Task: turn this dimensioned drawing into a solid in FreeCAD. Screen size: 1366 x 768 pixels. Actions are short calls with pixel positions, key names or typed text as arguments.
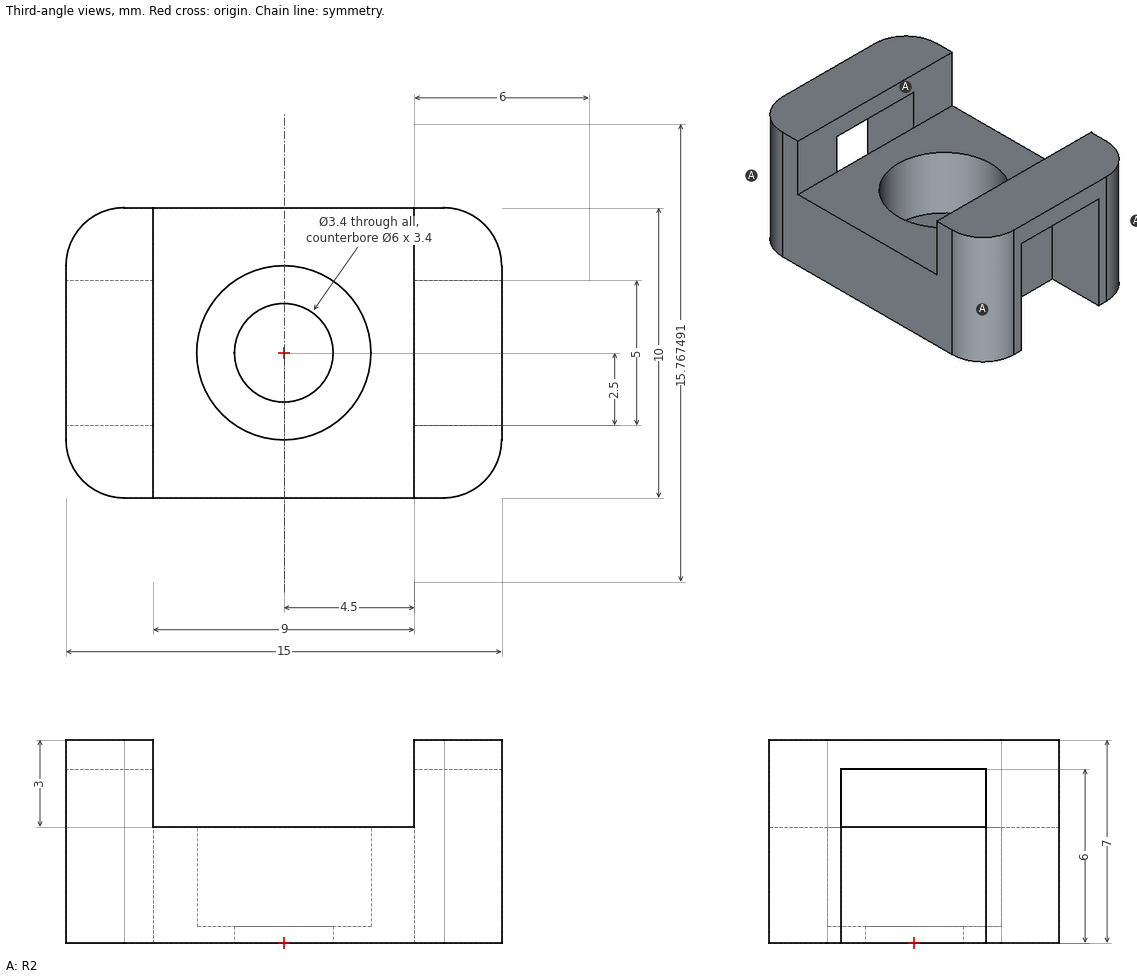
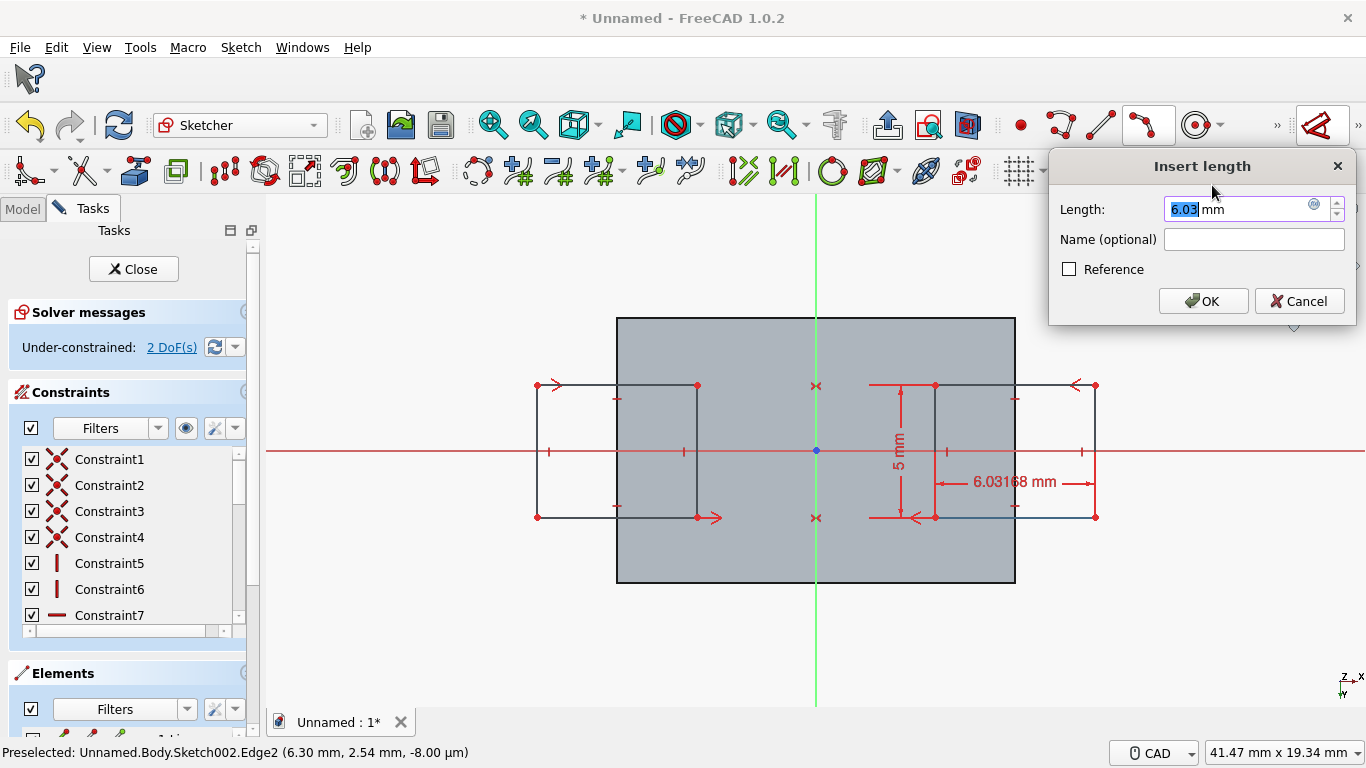
text(6)
key(Return)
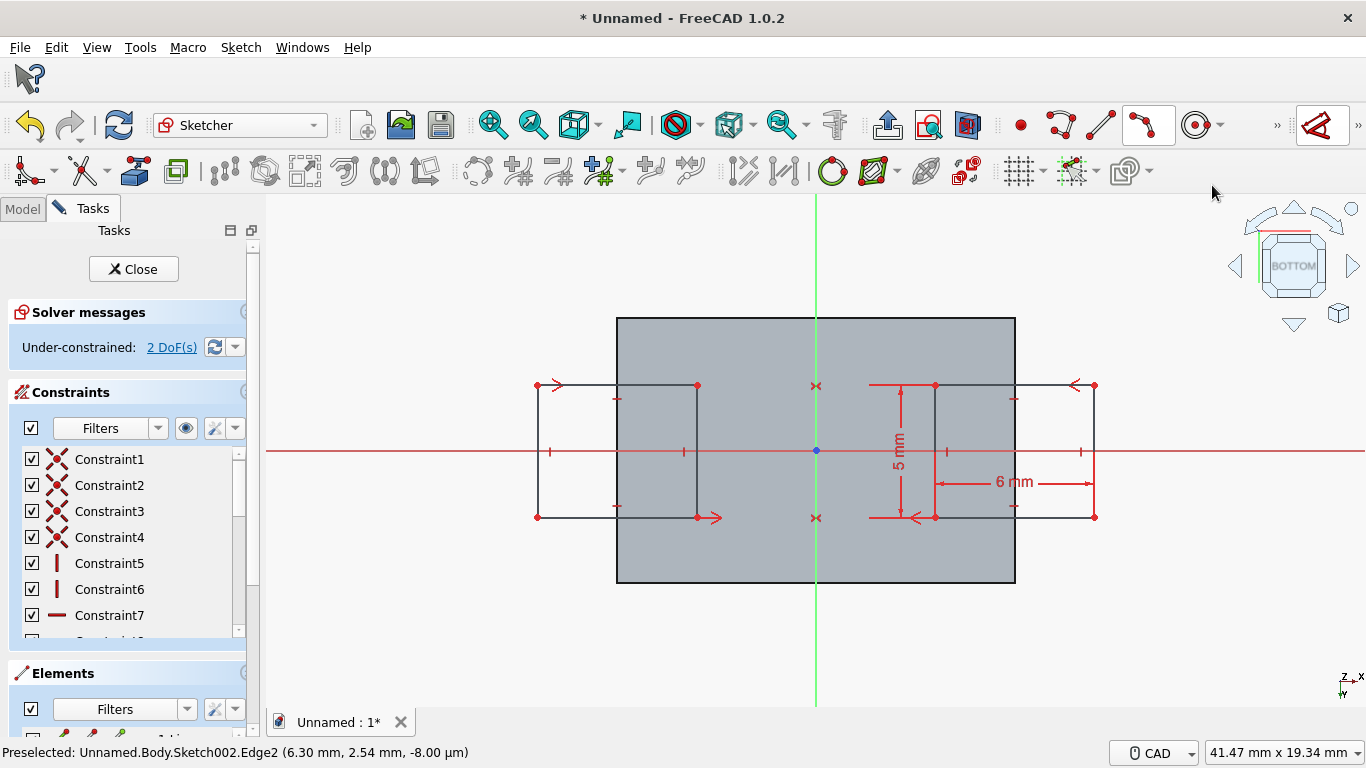
click(935, 385)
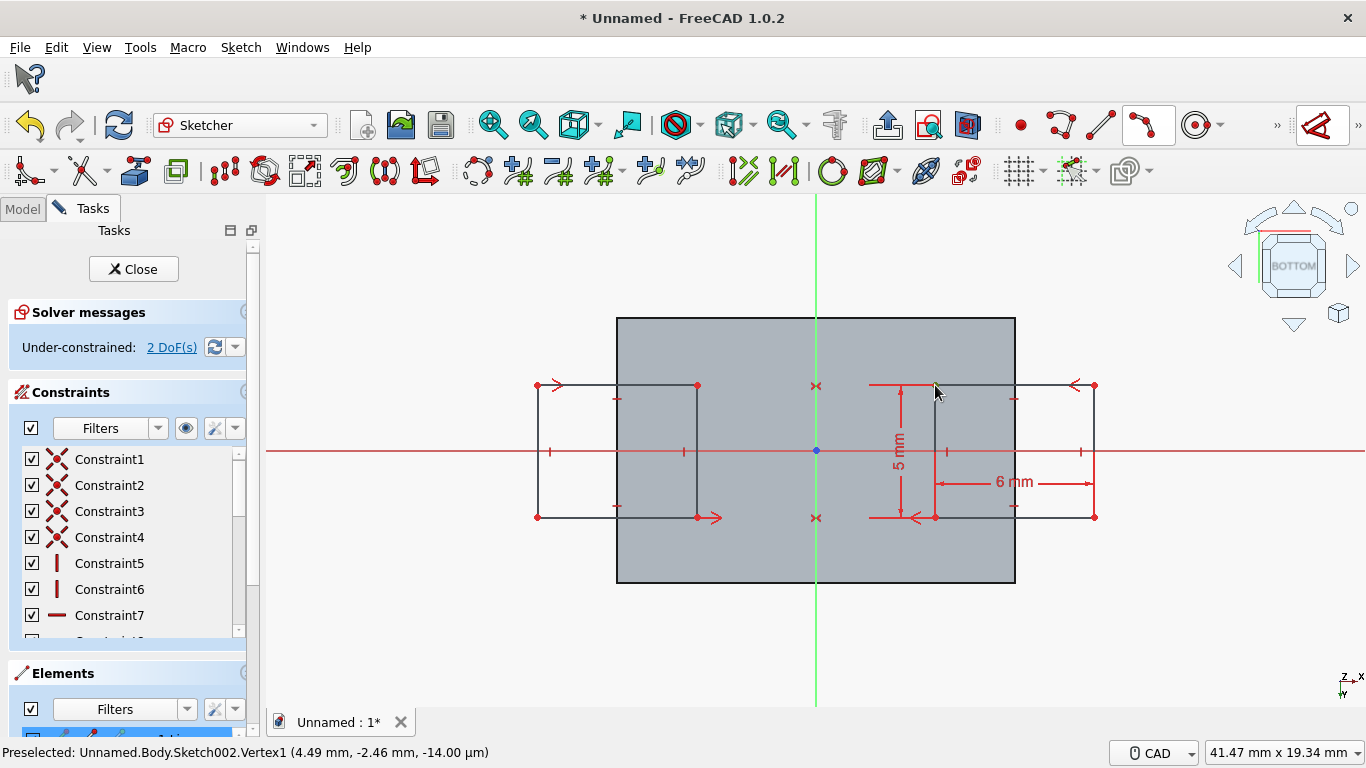
key(l)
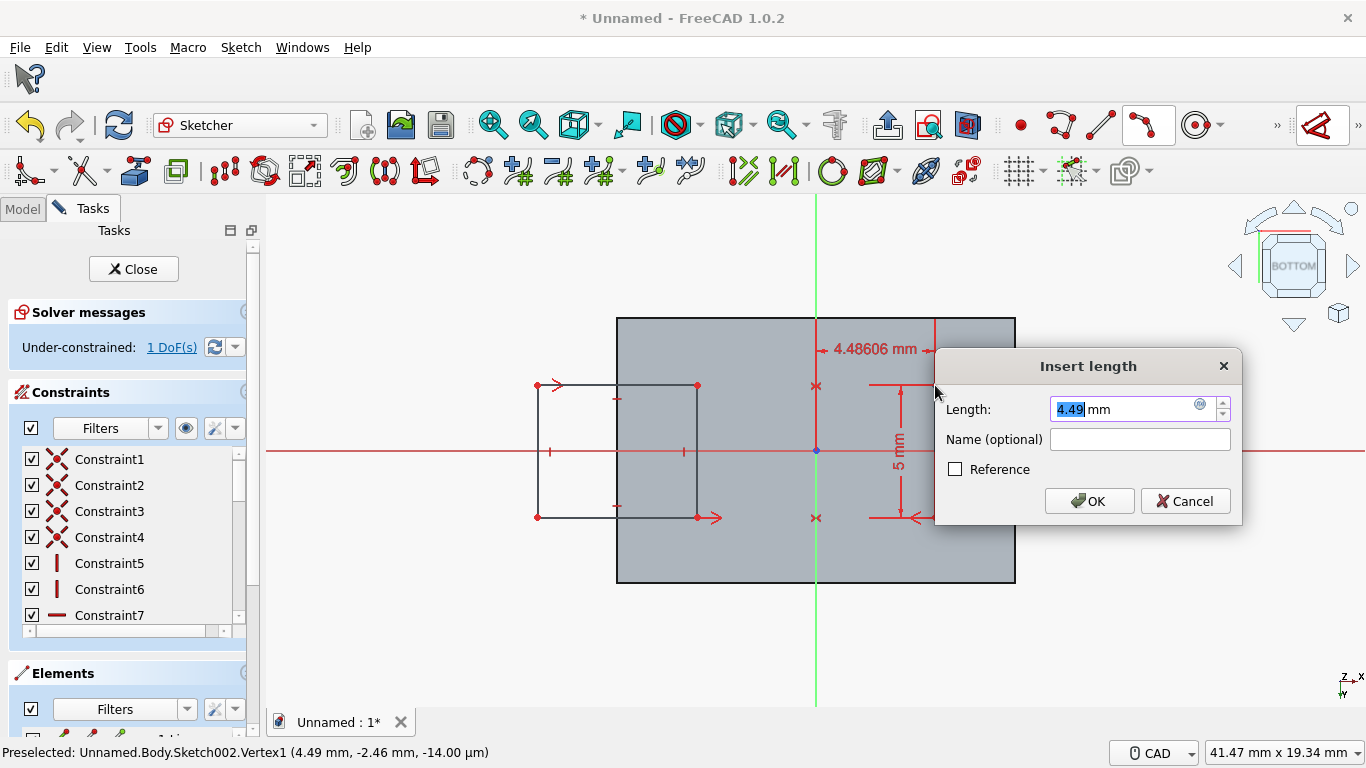
text(4.5)
key(Return)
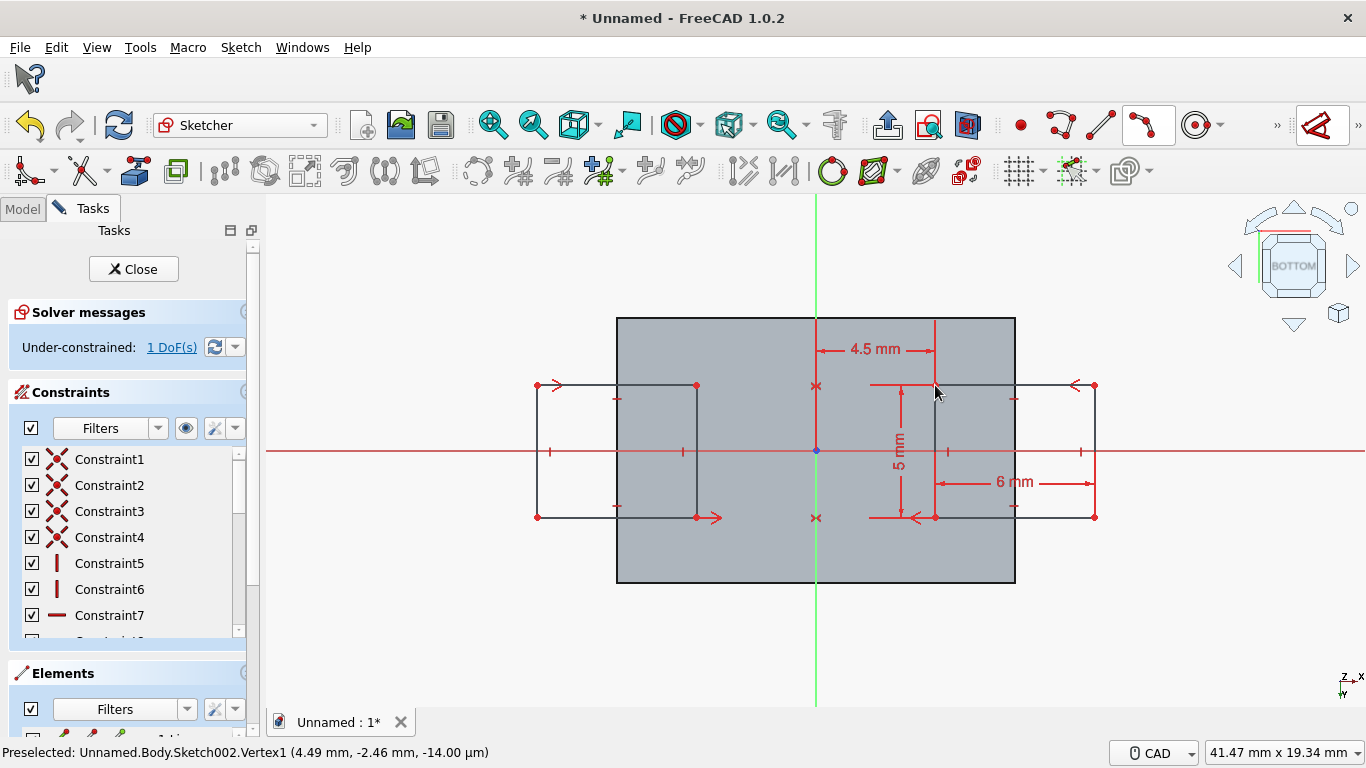
click(935, 385)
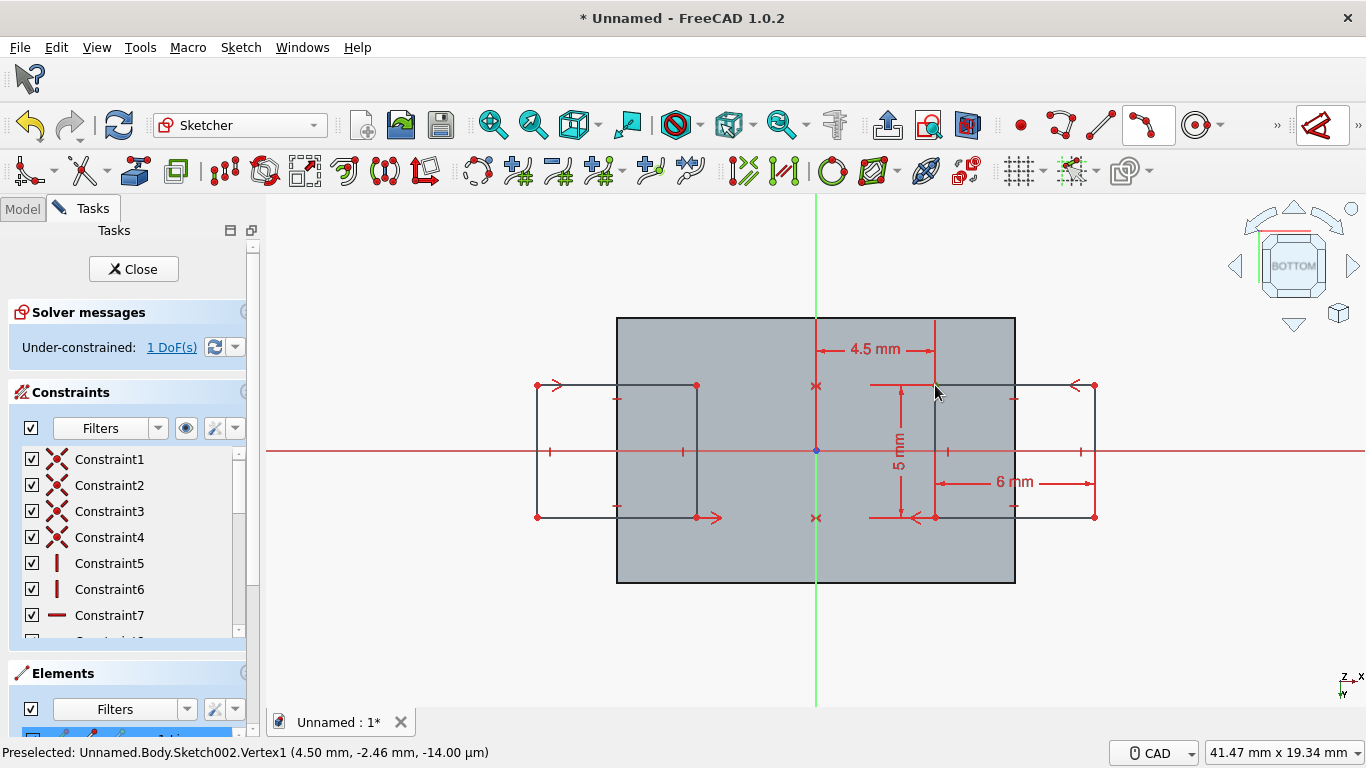
click(1344, 126)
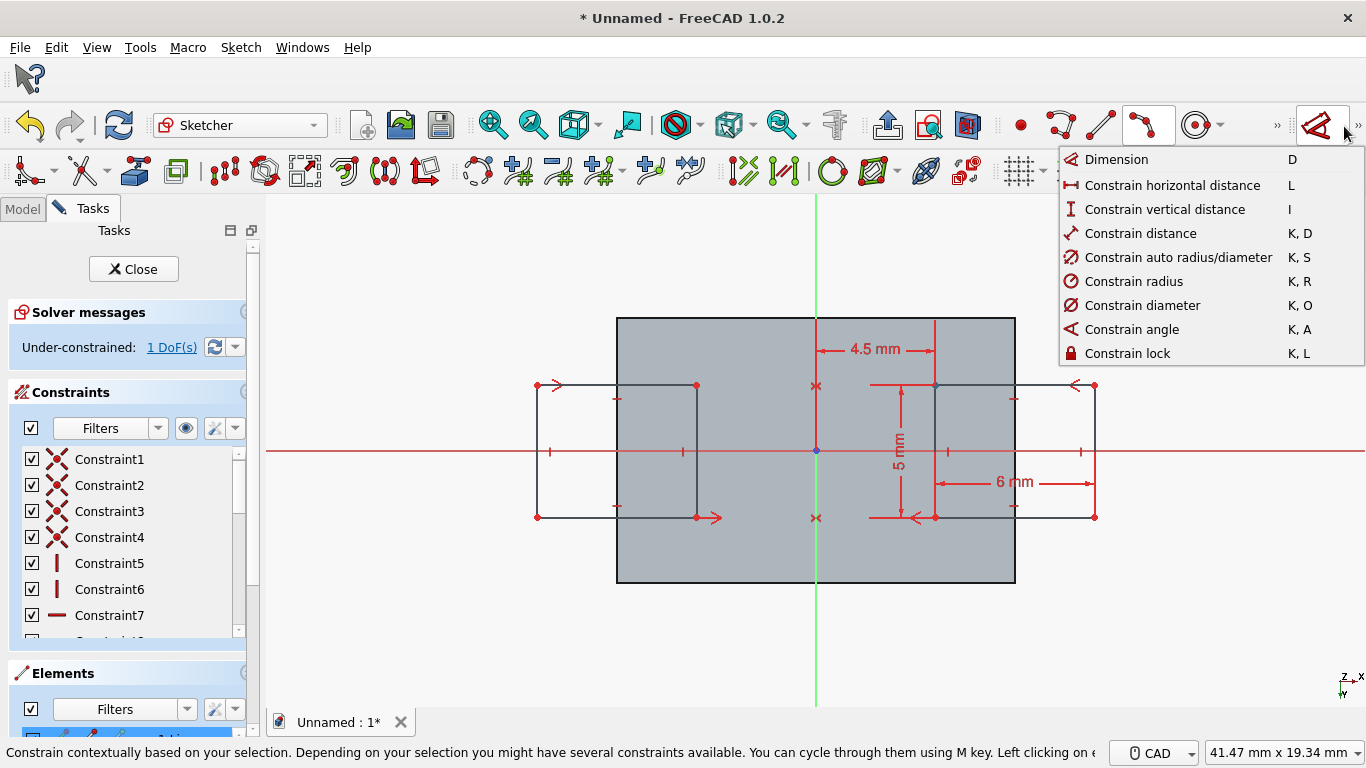
click(1212, 209)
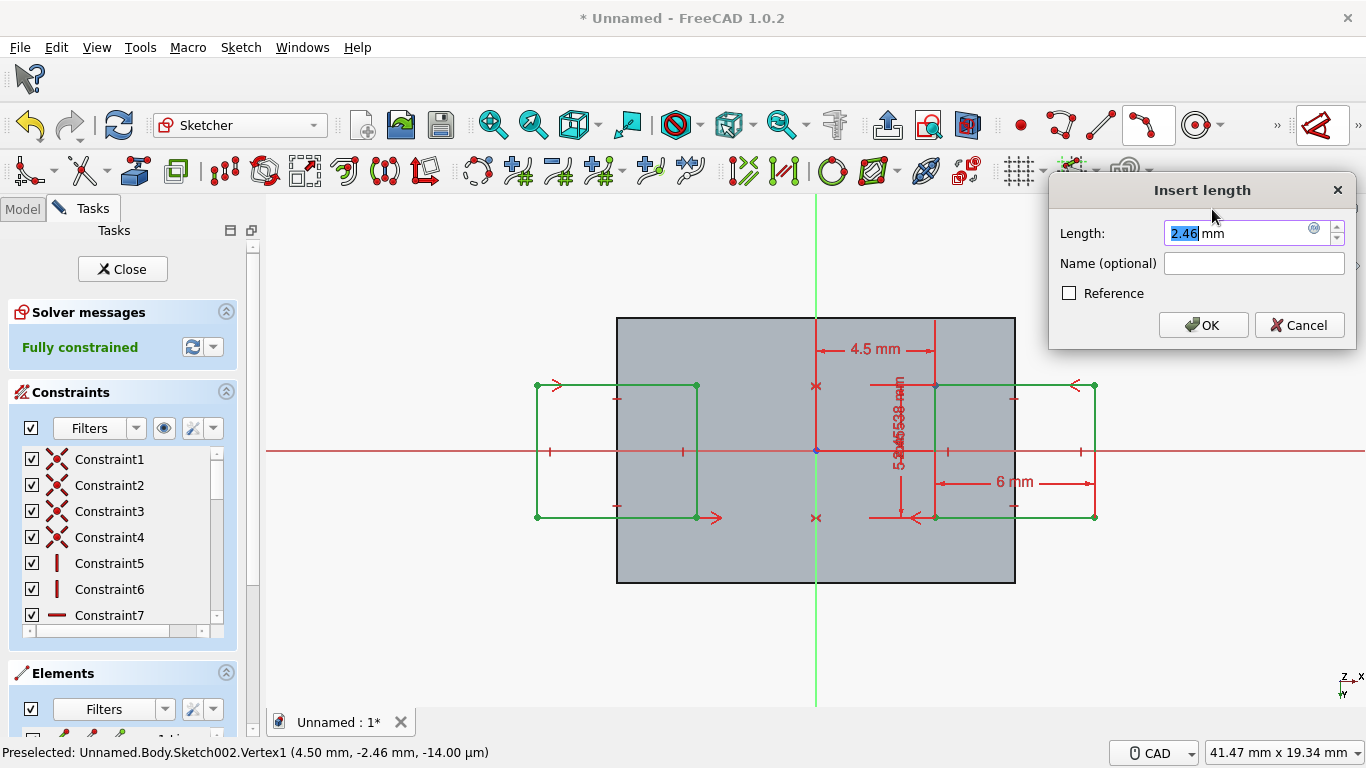
text(2.5)
key(Return)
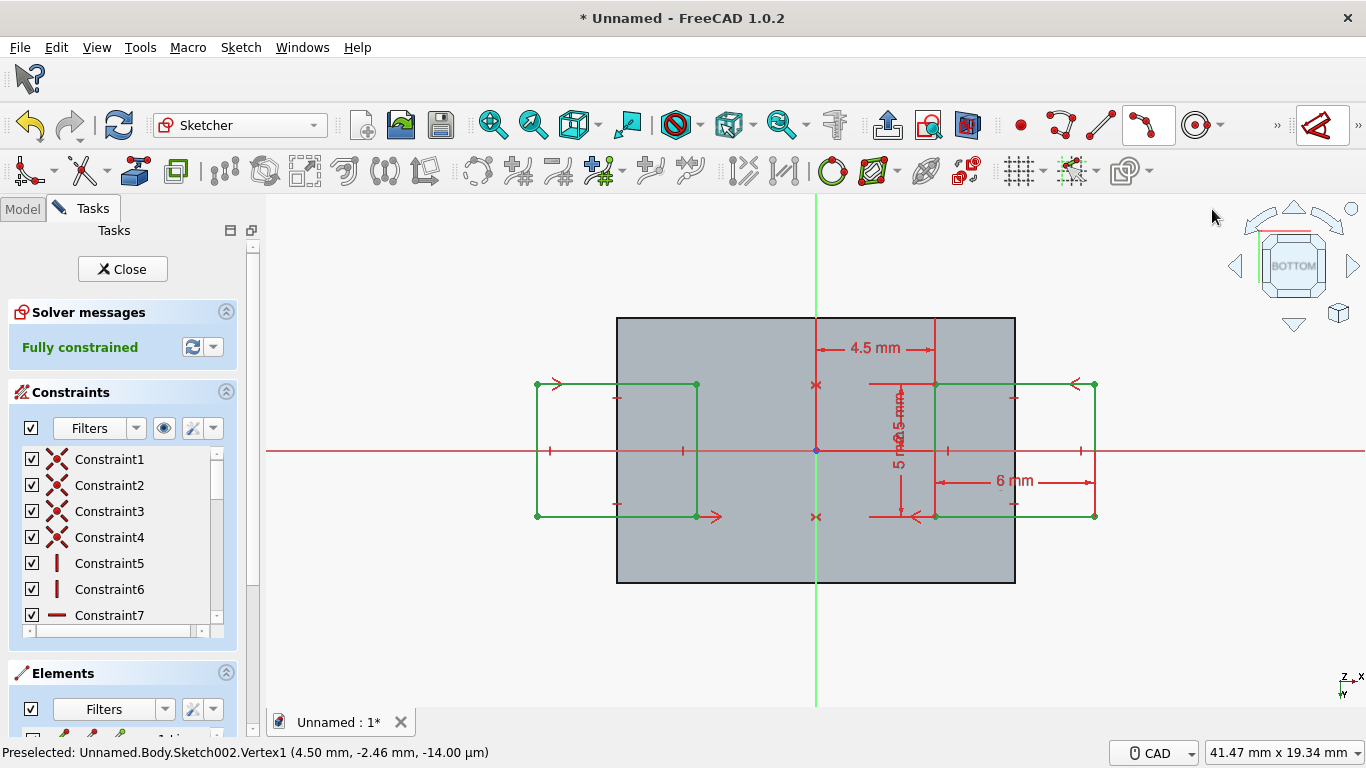
click(123, 269)